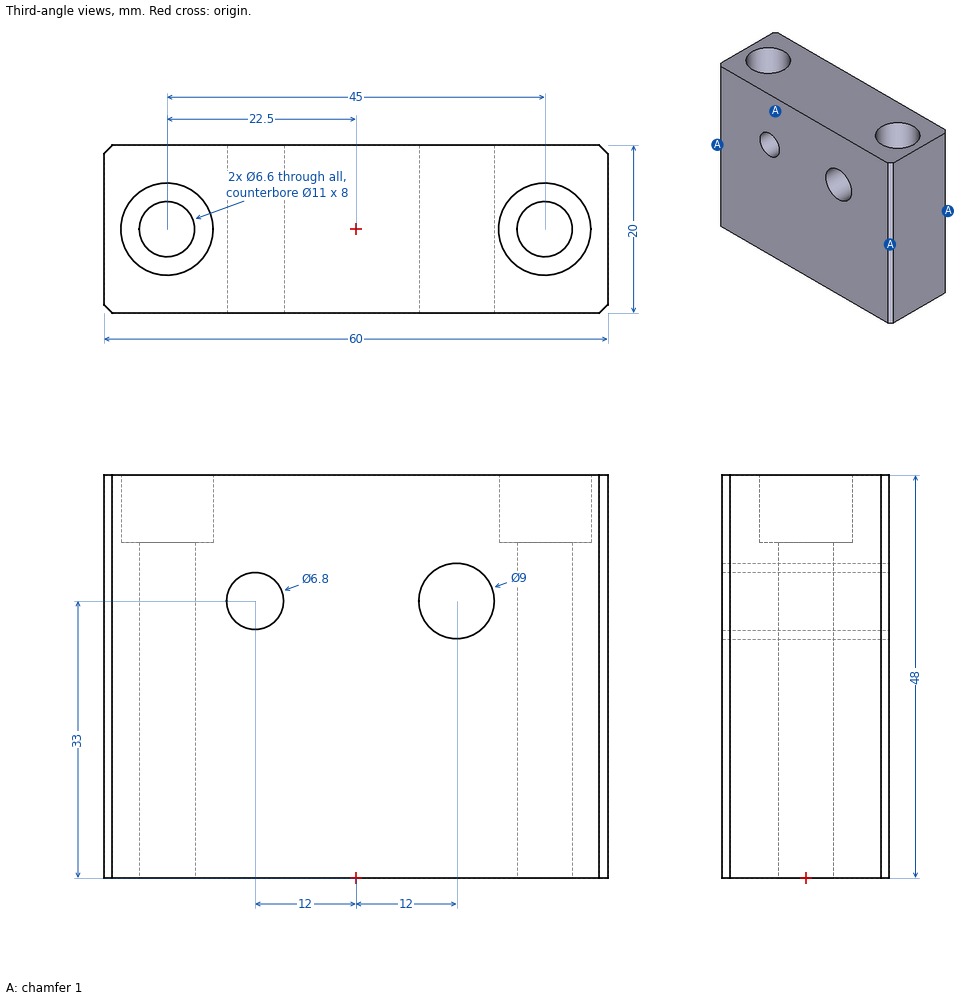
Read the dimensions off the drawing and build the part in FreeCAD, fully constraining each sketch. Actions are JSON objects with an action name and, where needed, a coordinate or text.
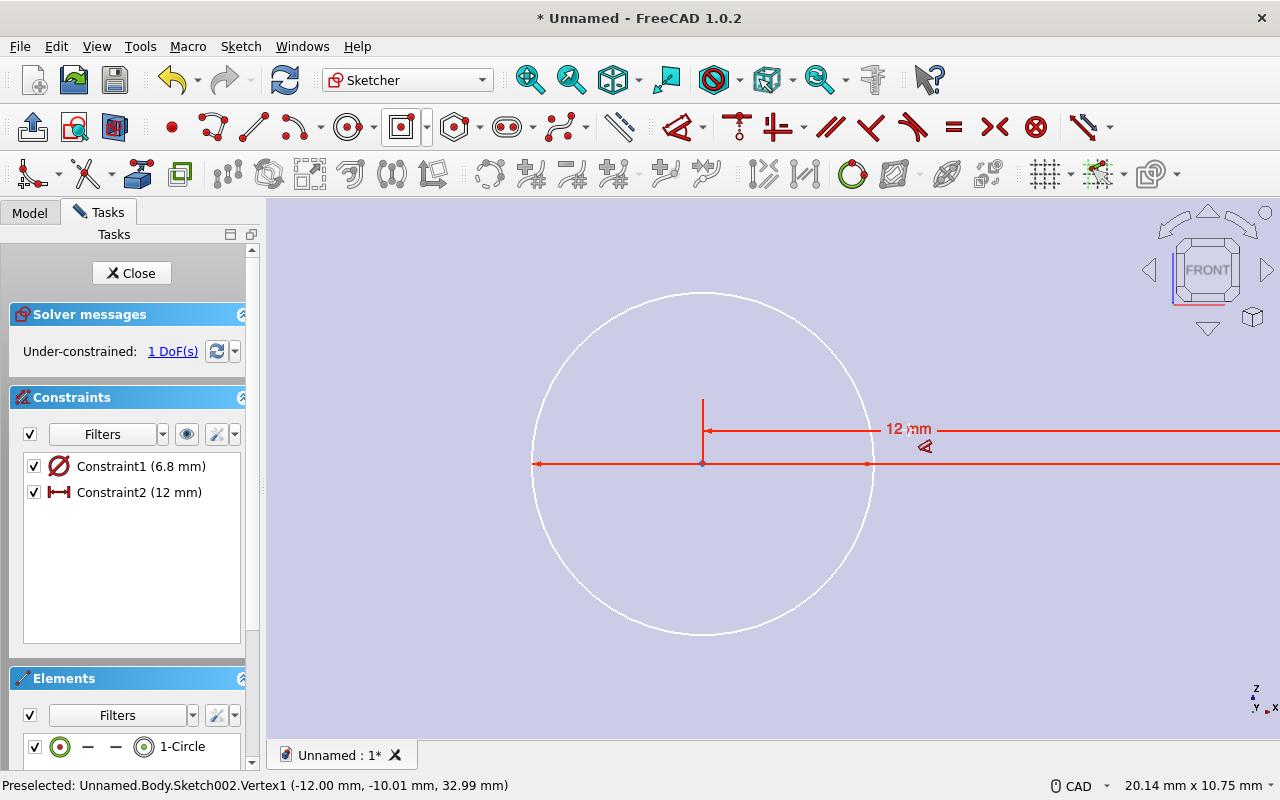
{"action": "left_click", "coordinate": [703, 464]}
{"action": "left_click", "coordinate": [669, 587]}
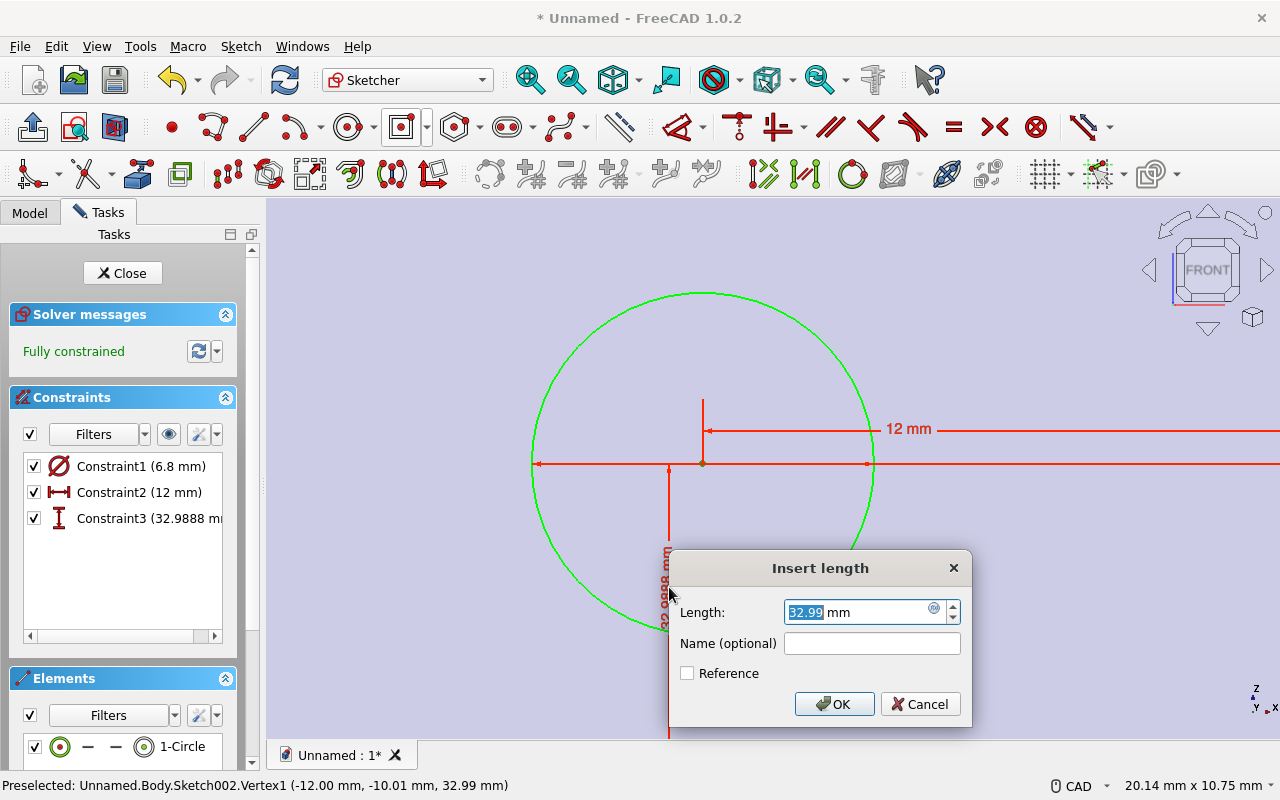
{"action": "type", "text": "33"}
{"action": "key", "text": "Return"}
{"action": "key", "text": "Escape"}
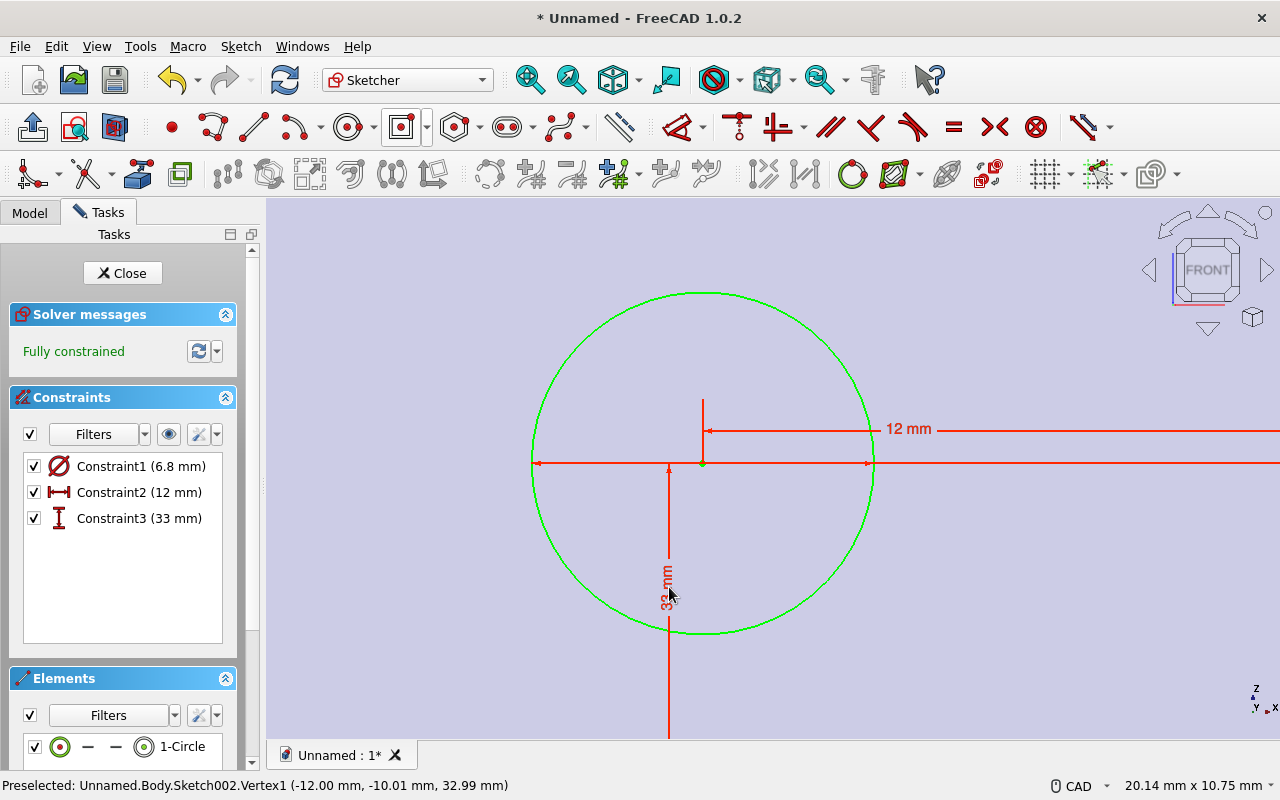
{"action": "left_click", "coordinate": [123, 273]}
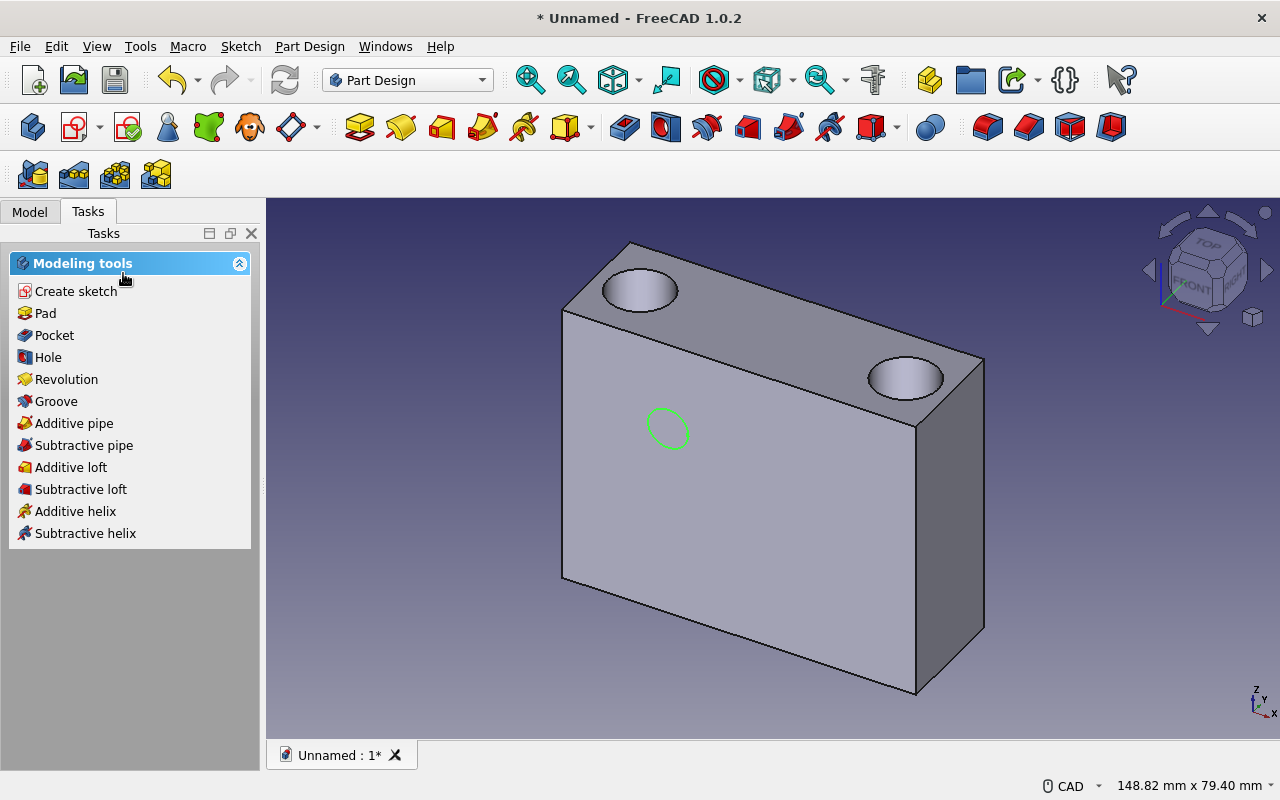
{"action": "left_click", "coordinate": [625, 128]}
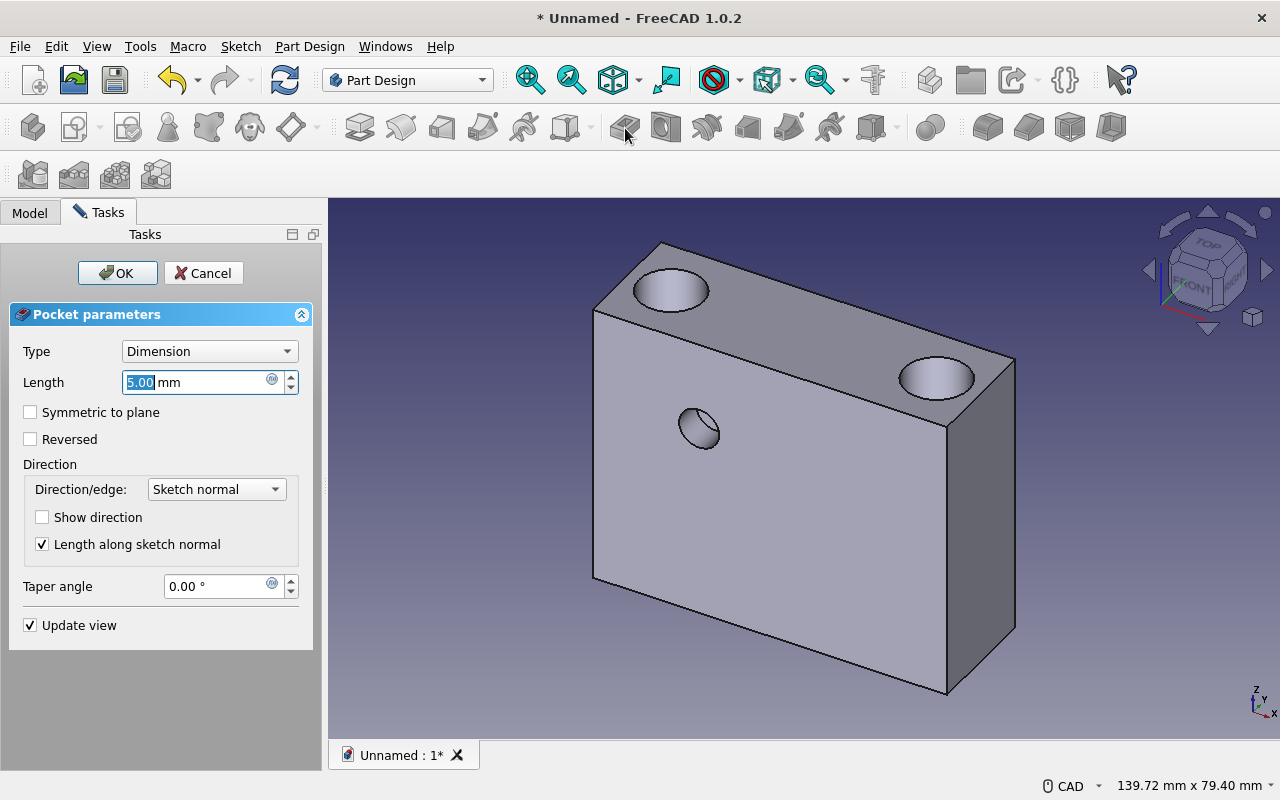
{"action": "left_click", "coordinate": [210, 352]}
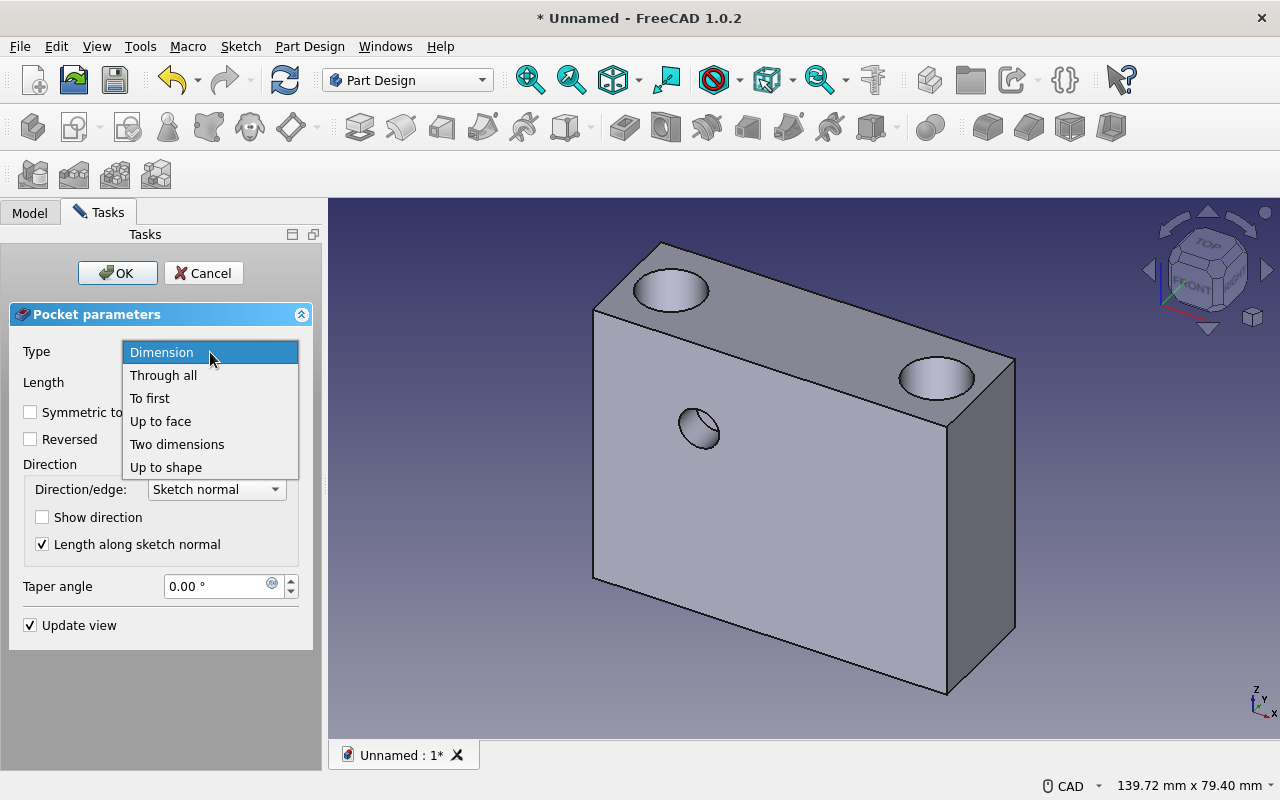
{"action": "left_click", "coordinate": [208, 376]}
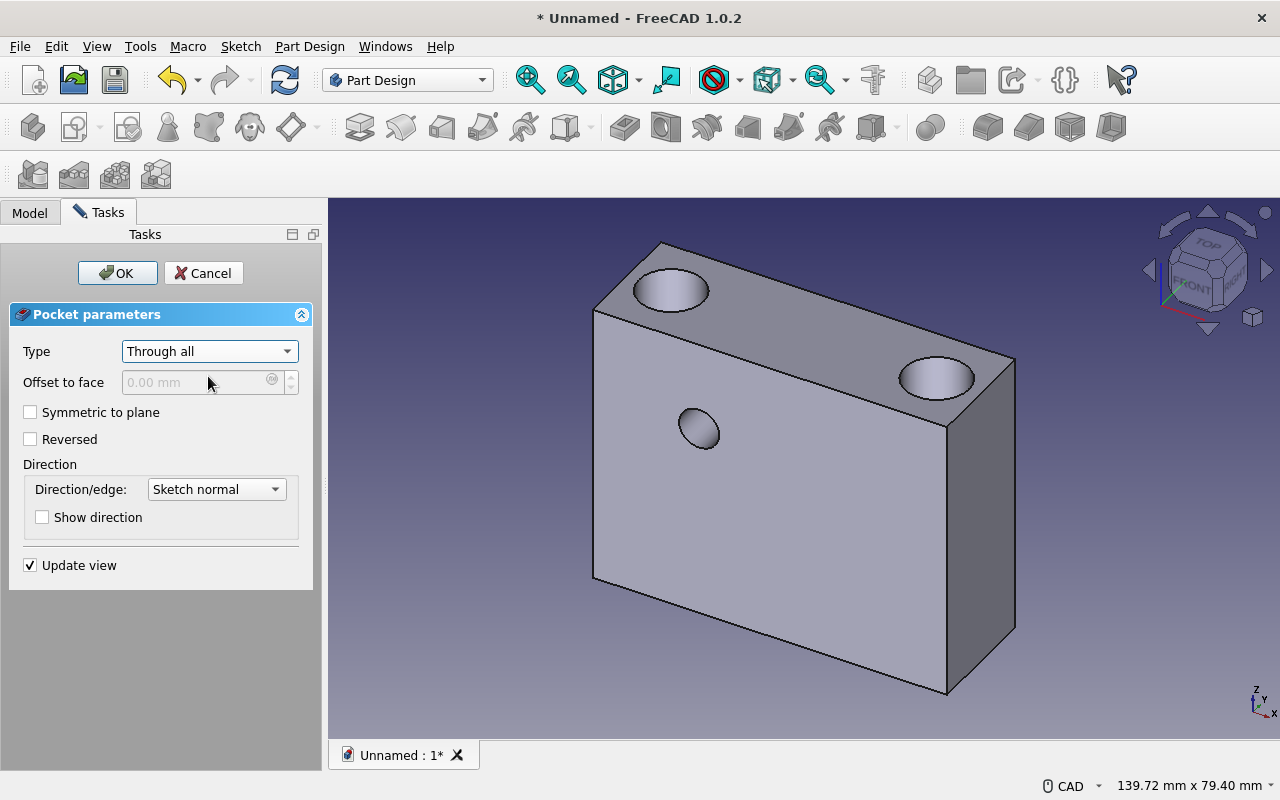
{"action": "left_click", "coordinate": [118, 273]}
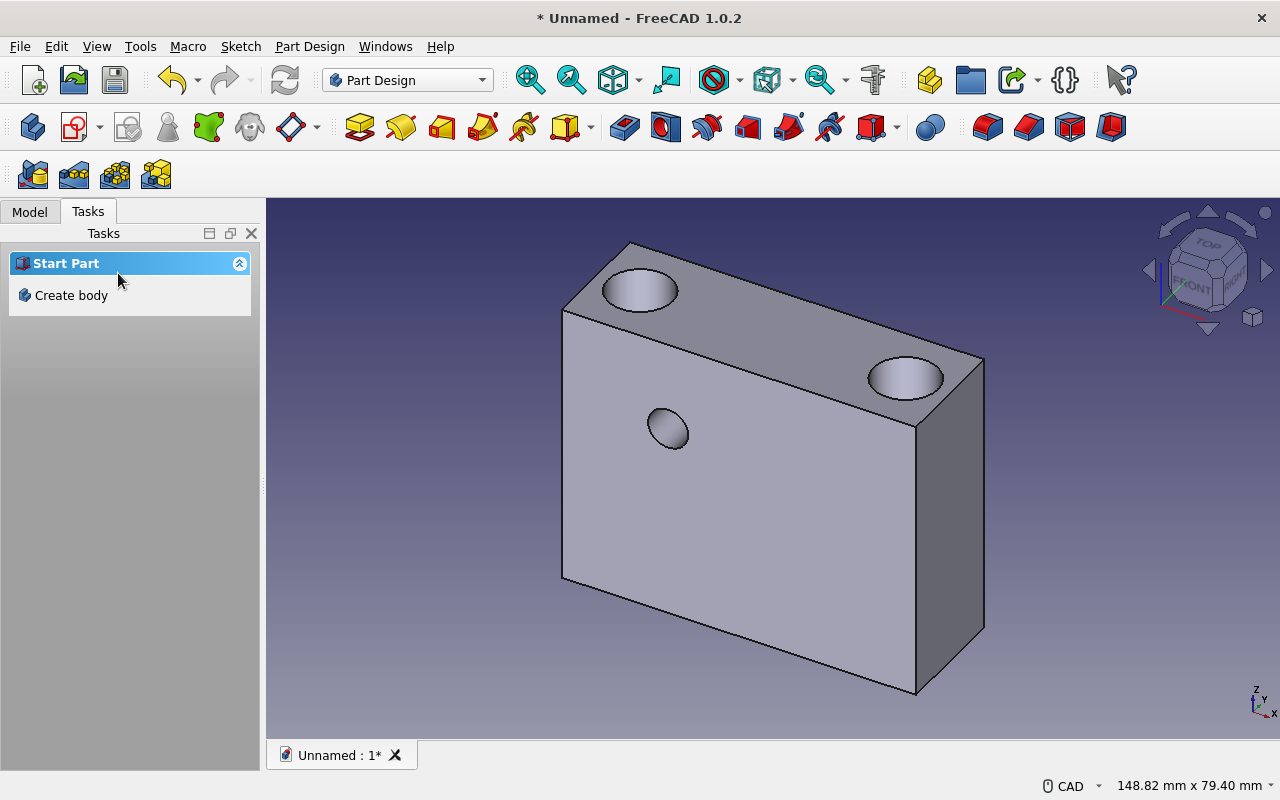
{"action": "left_click", "coordinate": [790, 518]}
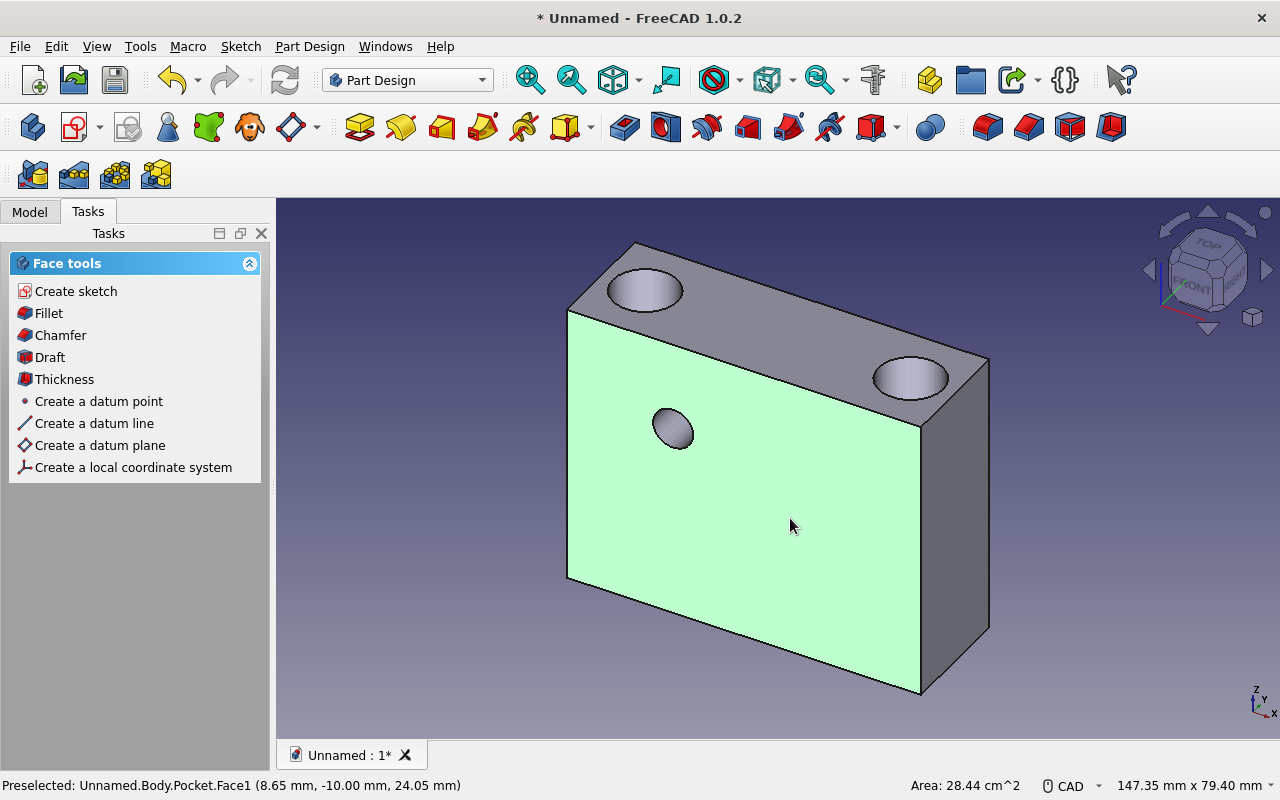
{"action": "left_click", "coordinate": [74, 128]}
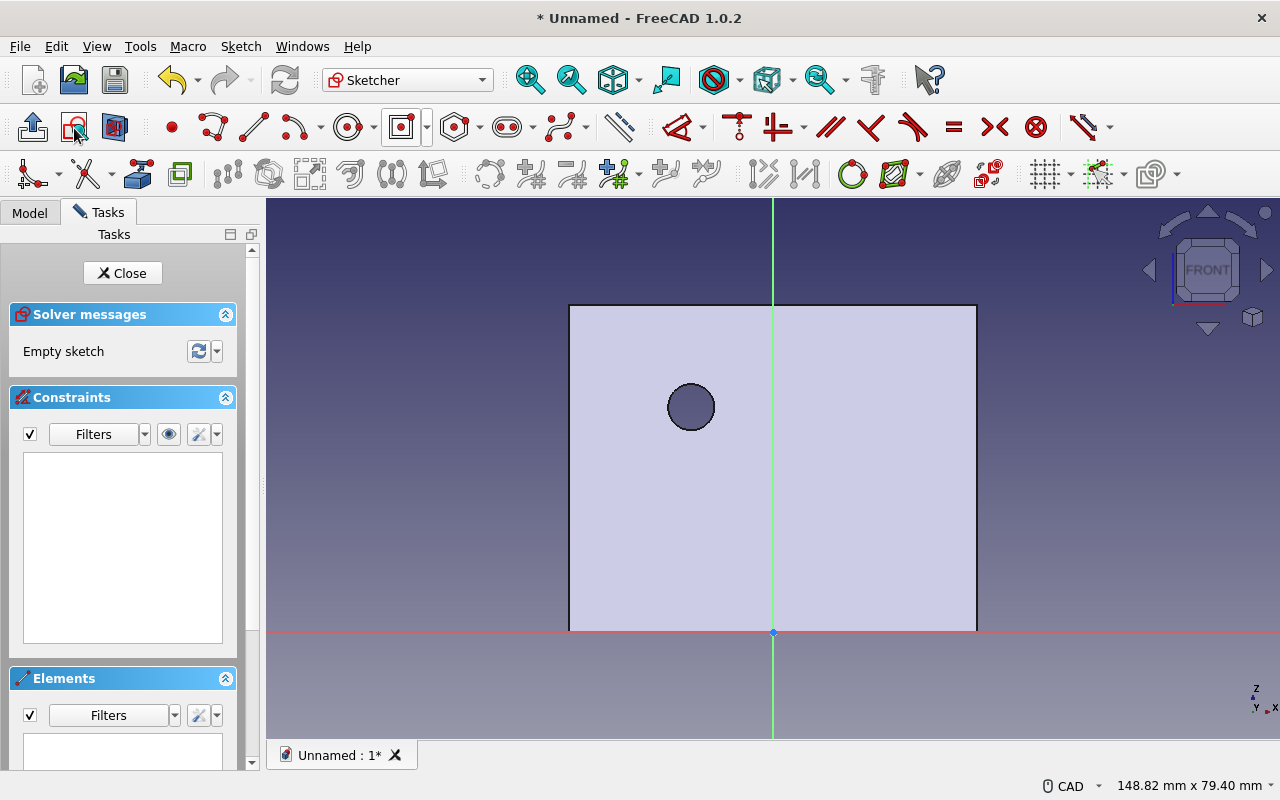
{"action": "scroll", "coordinate": [885, 395], "scroll_direction": "up", "scroll_amount": 9}